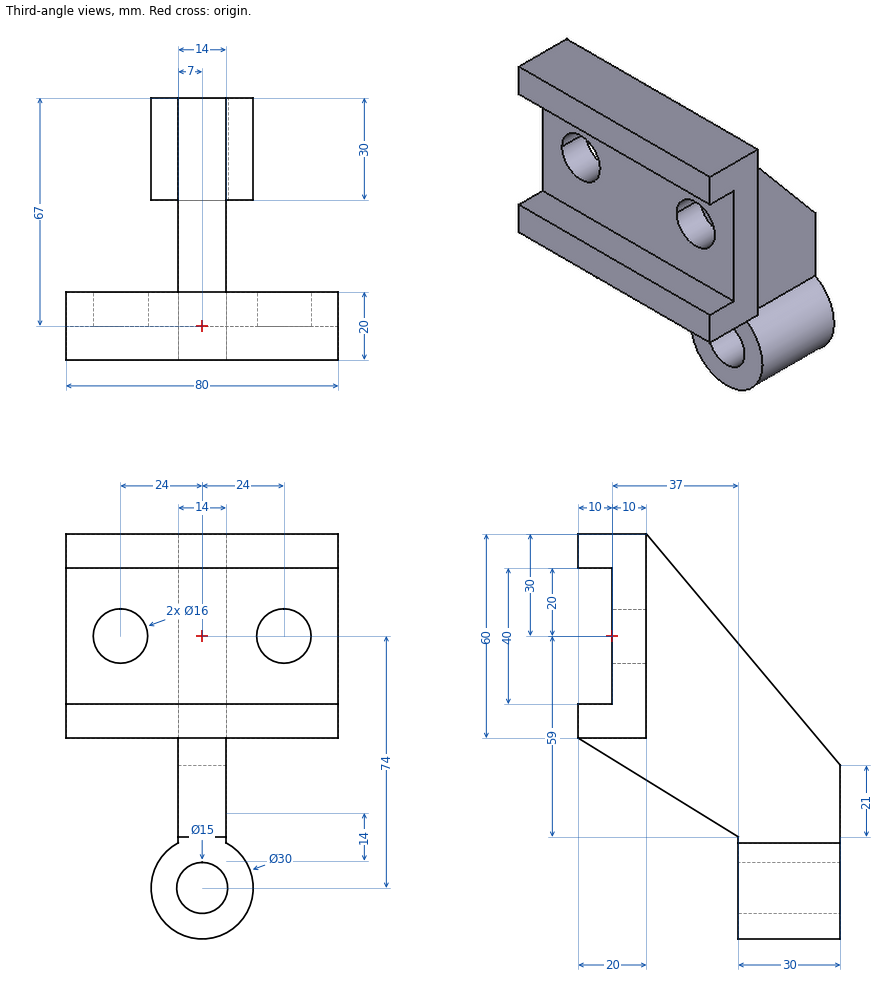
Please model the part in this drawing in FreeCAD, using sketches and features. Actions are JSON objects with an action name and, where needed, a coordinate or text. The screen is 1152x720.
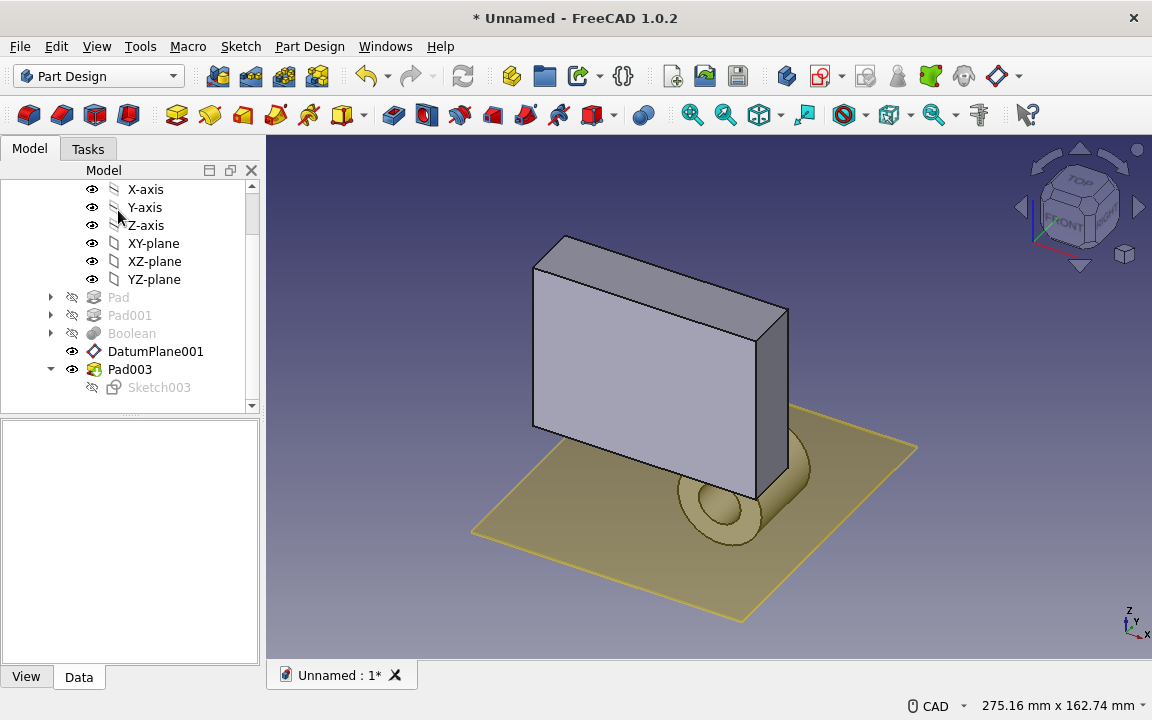
{"action": "left_click", "coordinate": [117, 351]}
{"action": "key", "text": "space"}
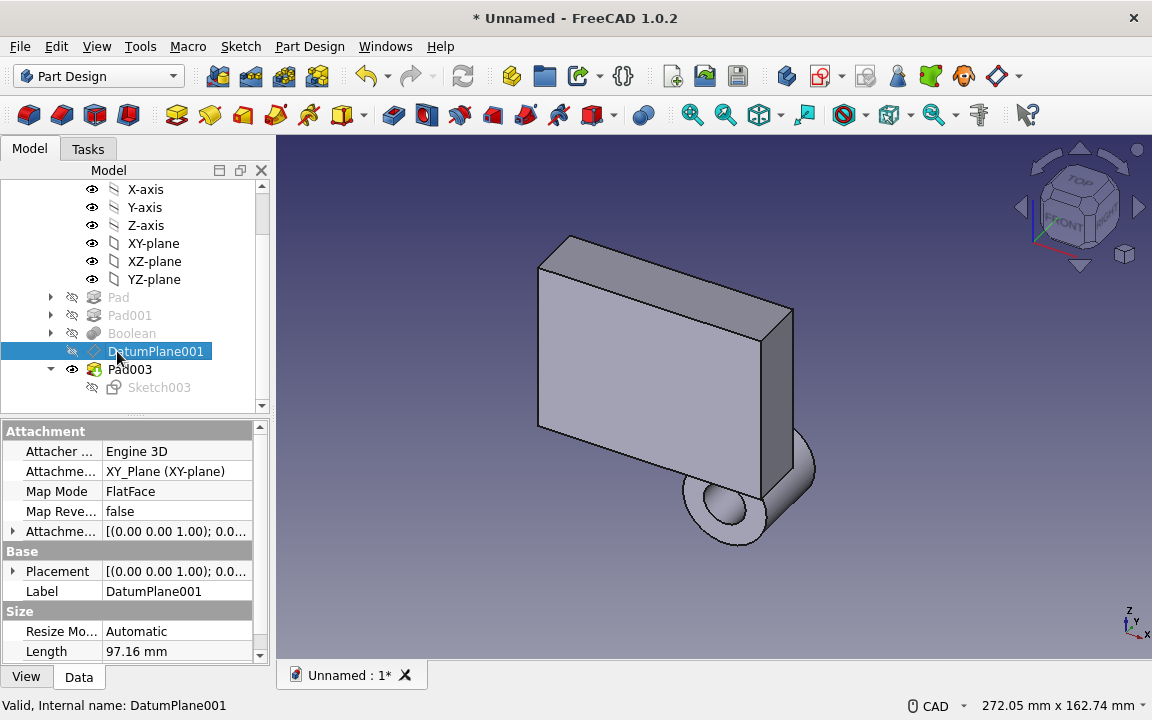
{"action": "left_click", "coordinate": [777, 358]}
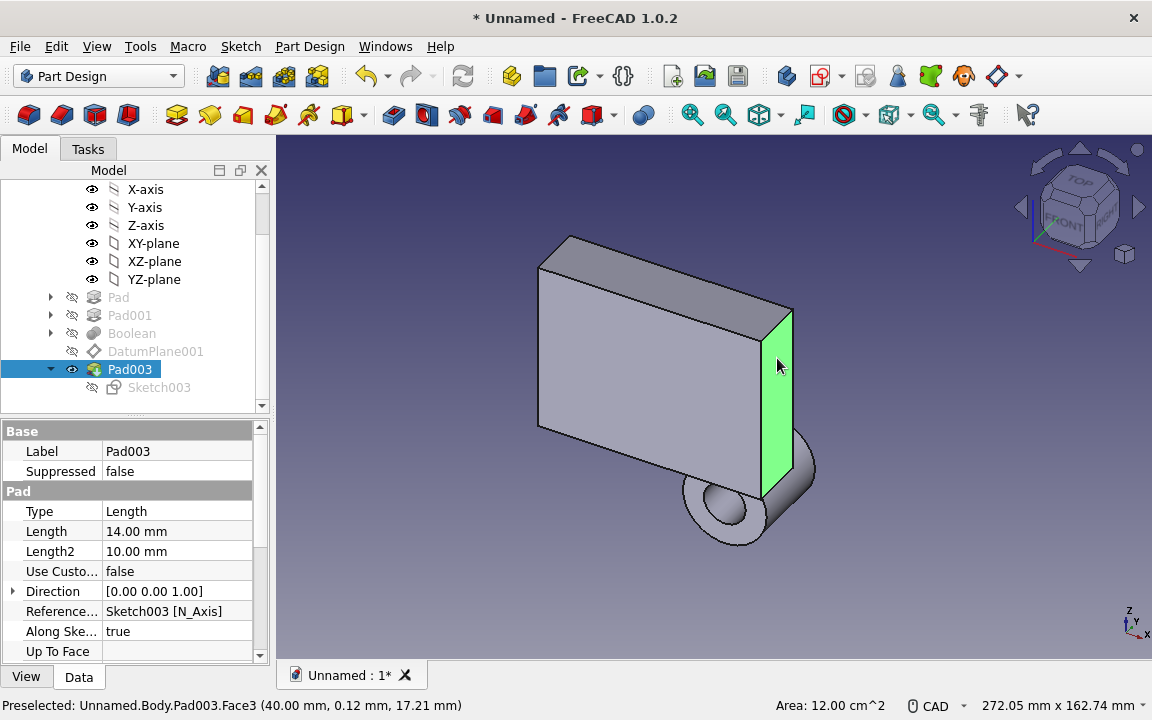
{"action": "left_click", "coordinate": [820, 76]}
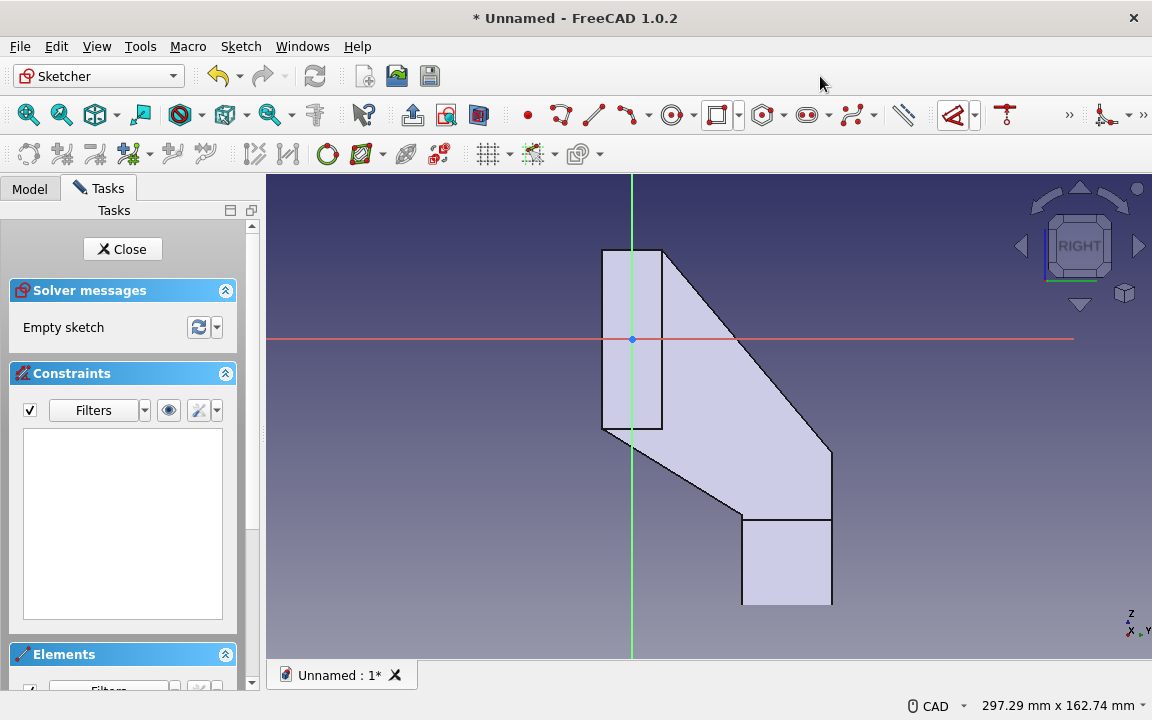
{"action": "scroll", "coordinate": [604, 295], "scroll_direction": "up", "scroll_amount": 5}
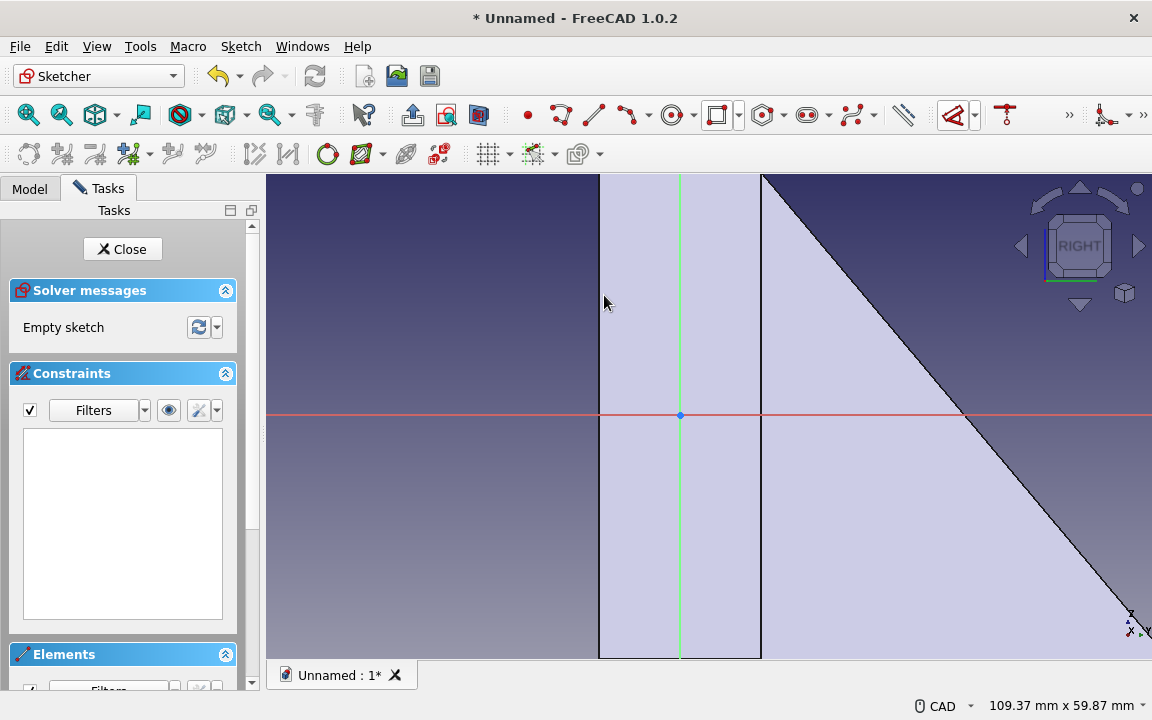
{"action": "left_click", "coordinate": [716, 116]}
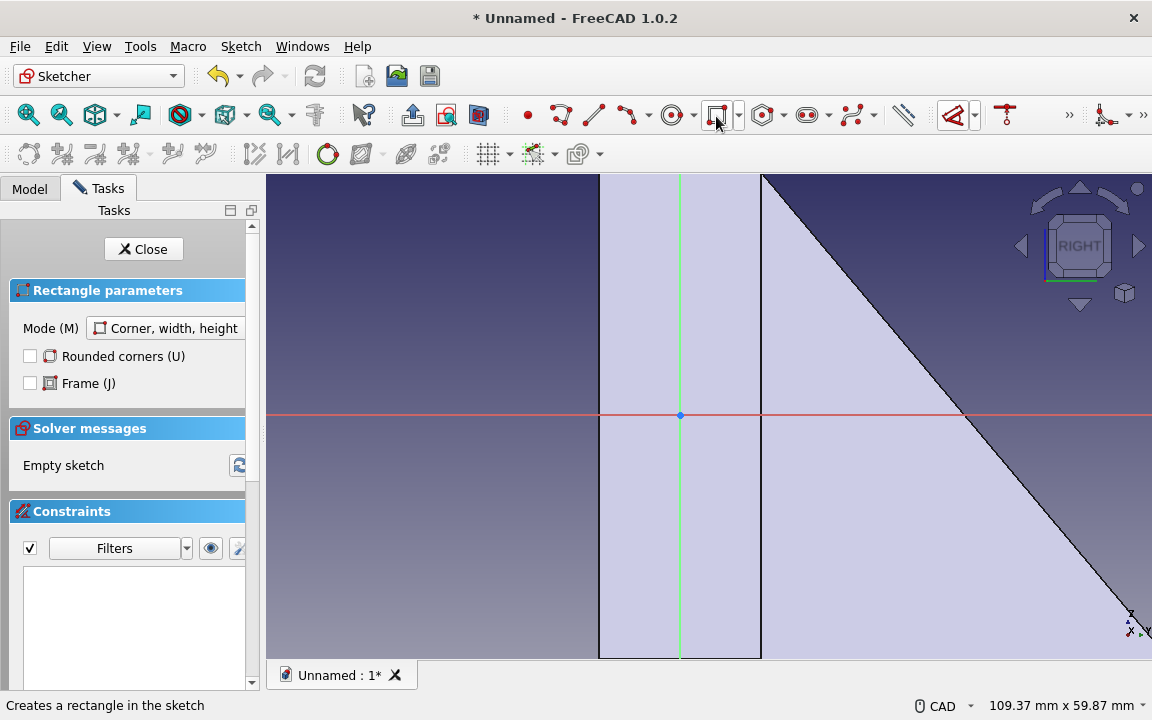
{"action": "left_click", "coordinate": [599, 253]}
{"action": "left_click", "coordinate": [680, 578]}
{"action": "key", "text": "Escape"}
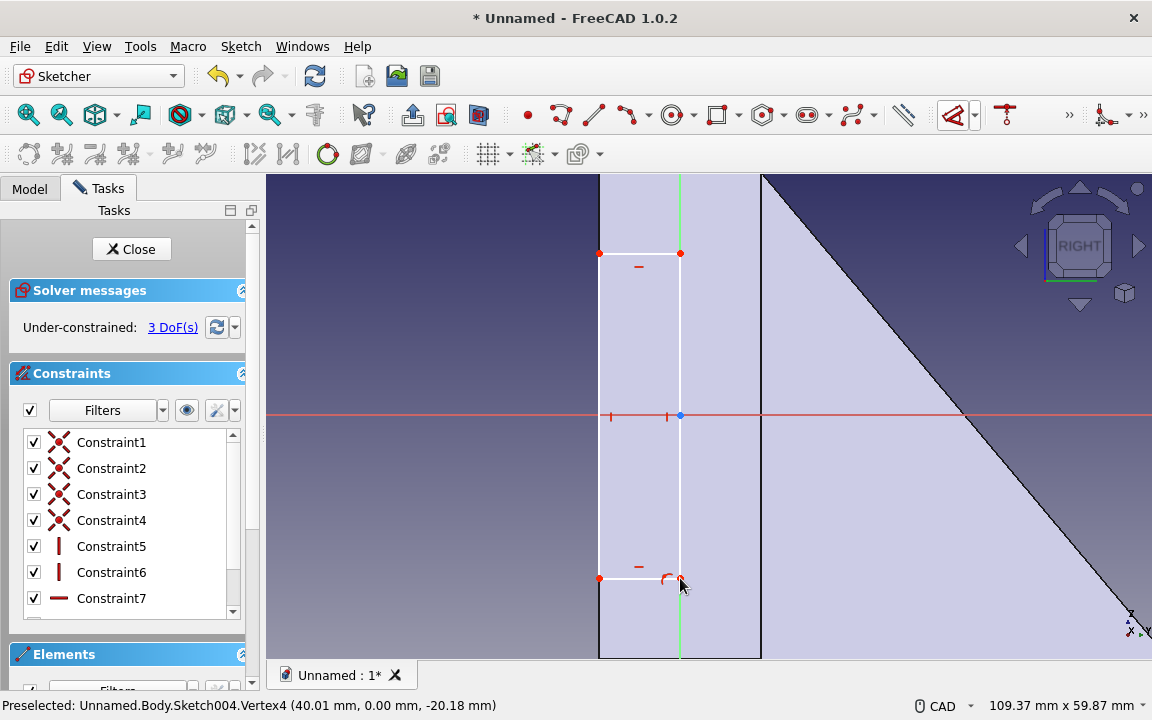
{"action": "left_click", "coordinate": [599, 351]}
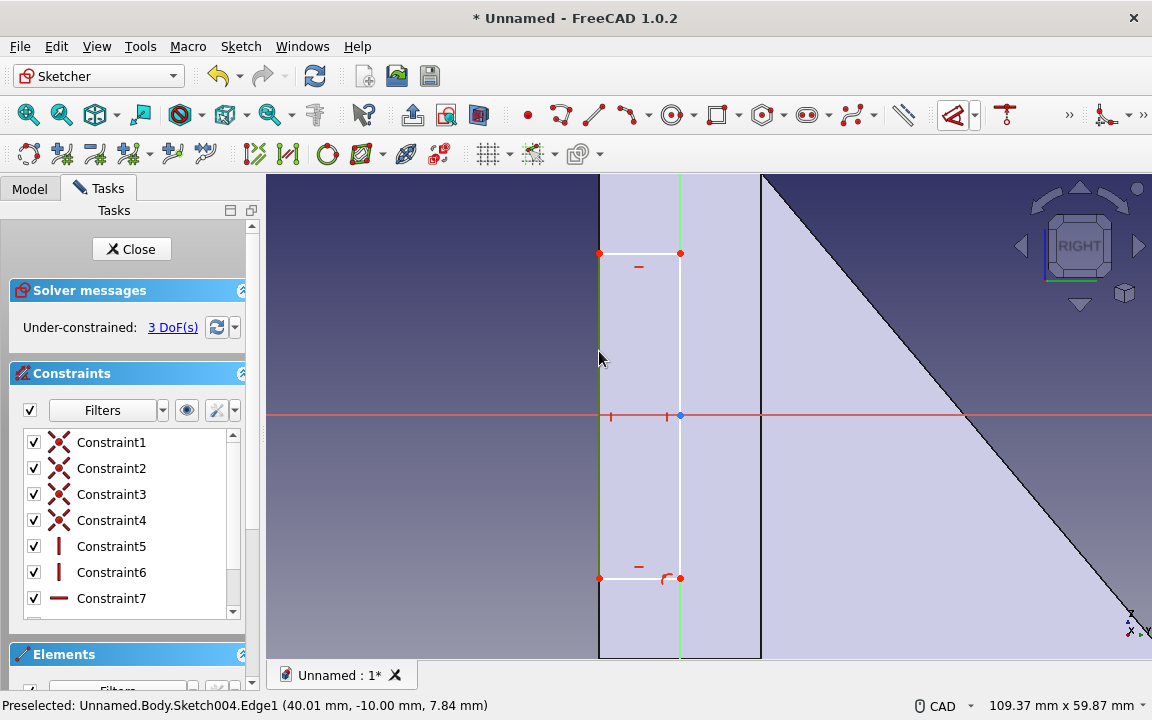
{"action": "key", "text": "i"}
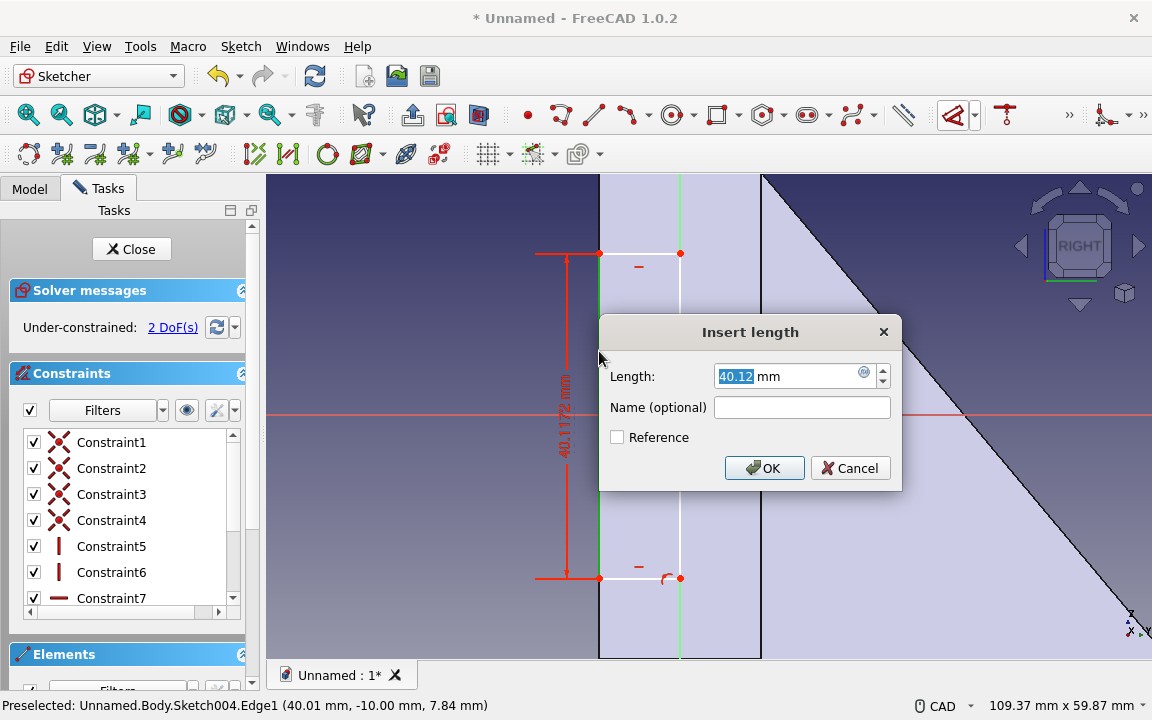
{"action": "type", "text": "40"}
{"action": "key", "text": "Return"}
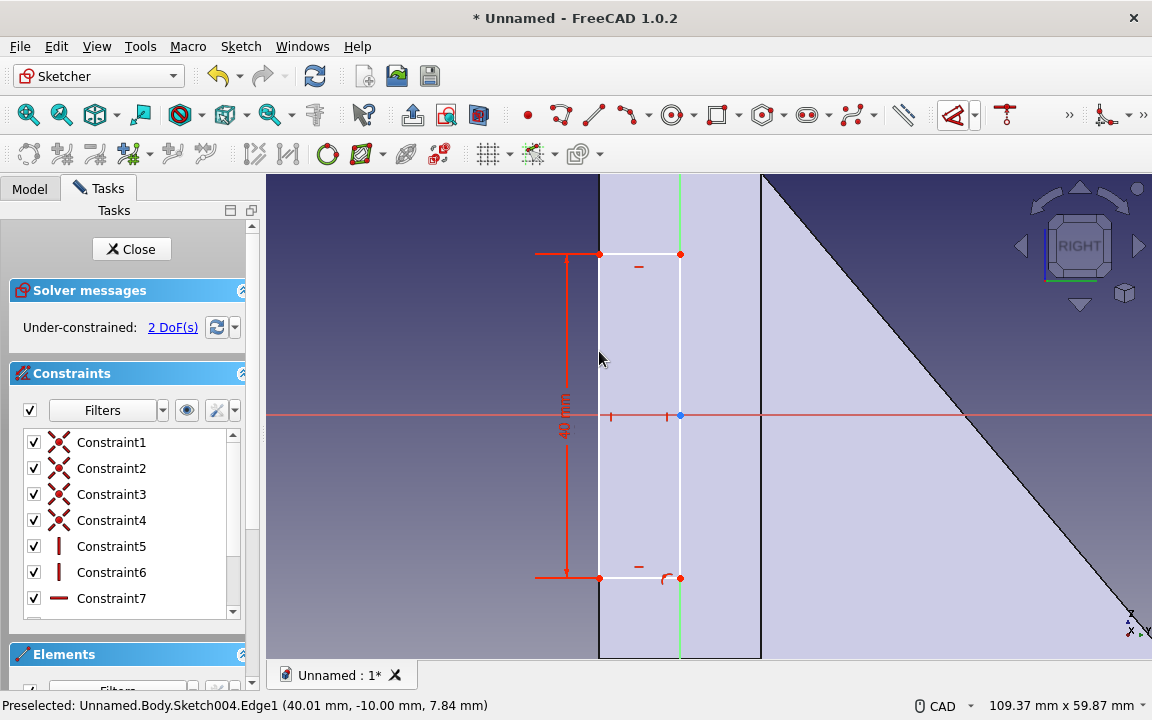
{"action": "left_click", "coordinate": [623, 578]}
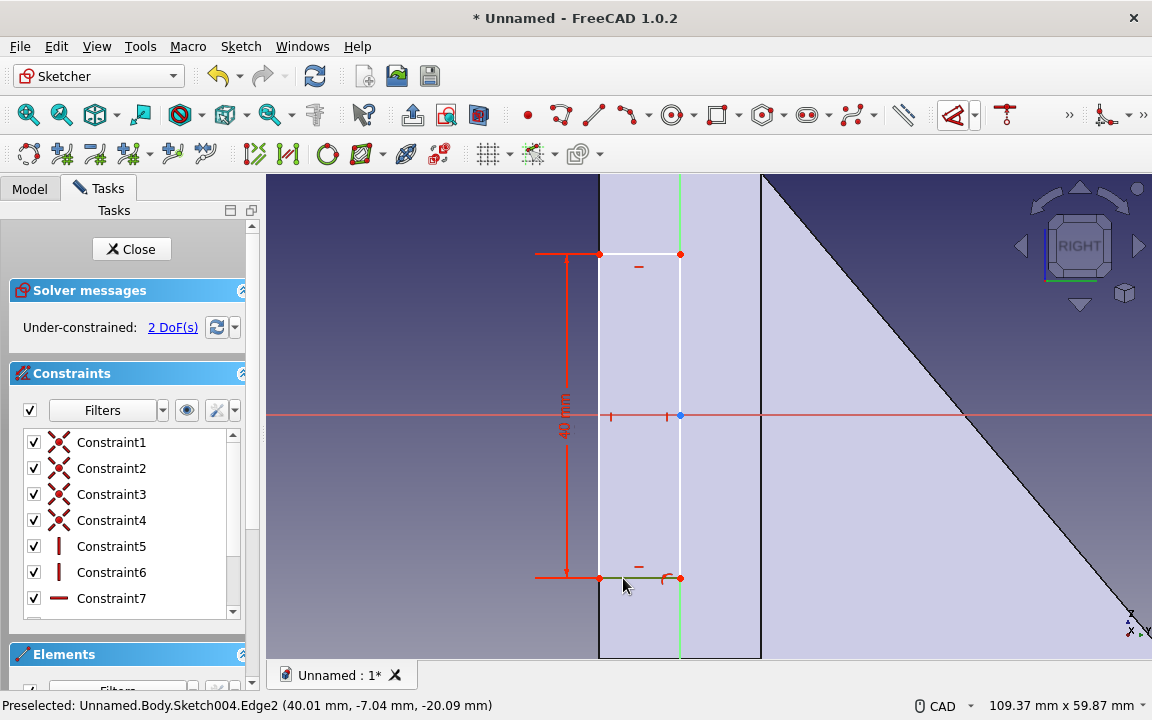
{"action": "left_click", "coordinate": [974, 116]}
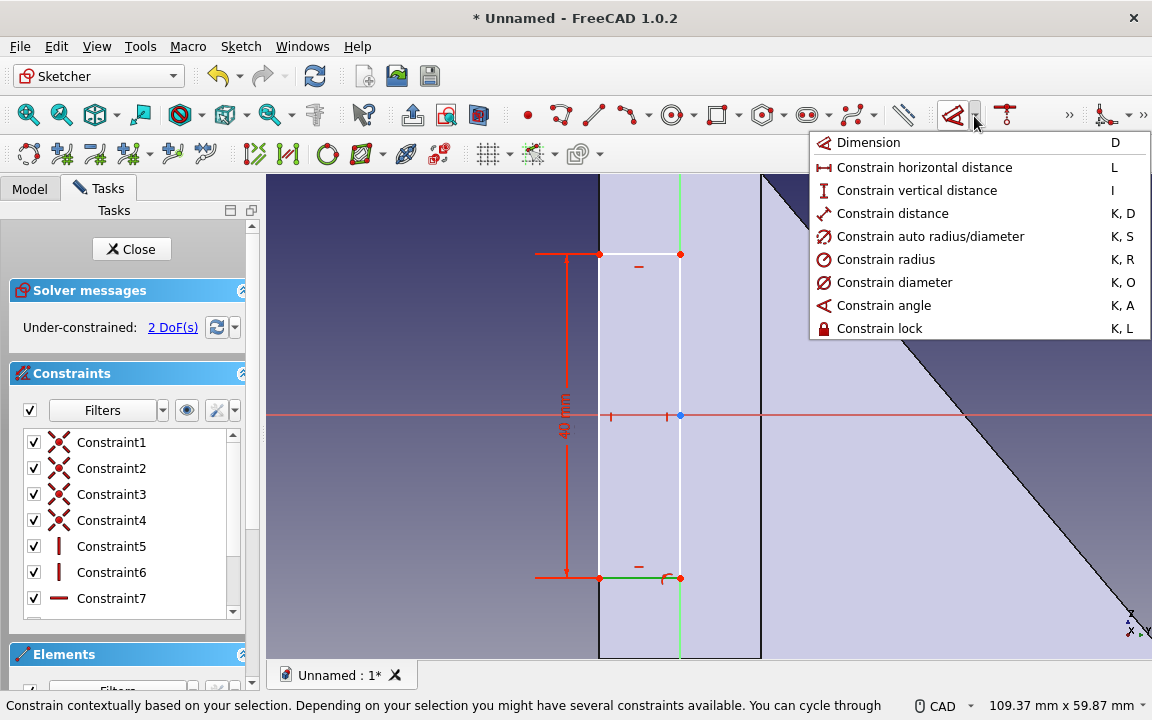
{"action": "left_click", "coordinate": [980, 168]}